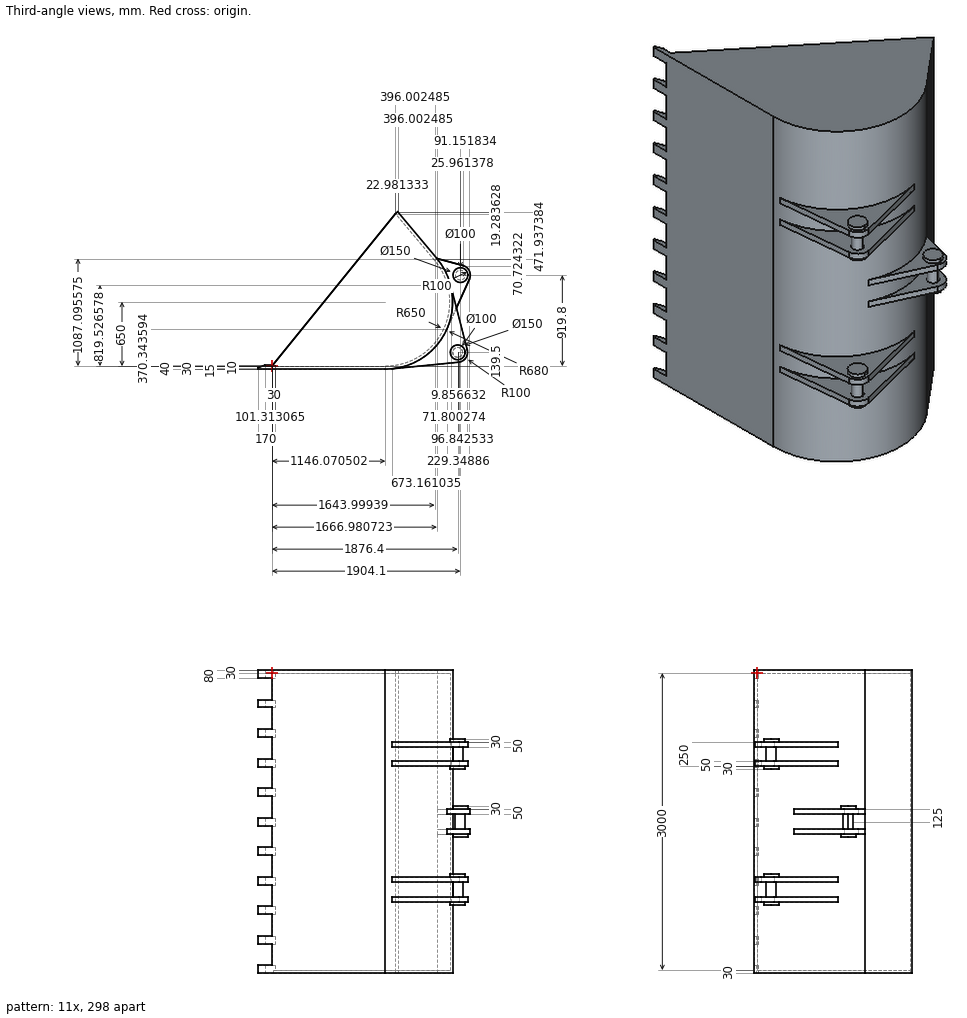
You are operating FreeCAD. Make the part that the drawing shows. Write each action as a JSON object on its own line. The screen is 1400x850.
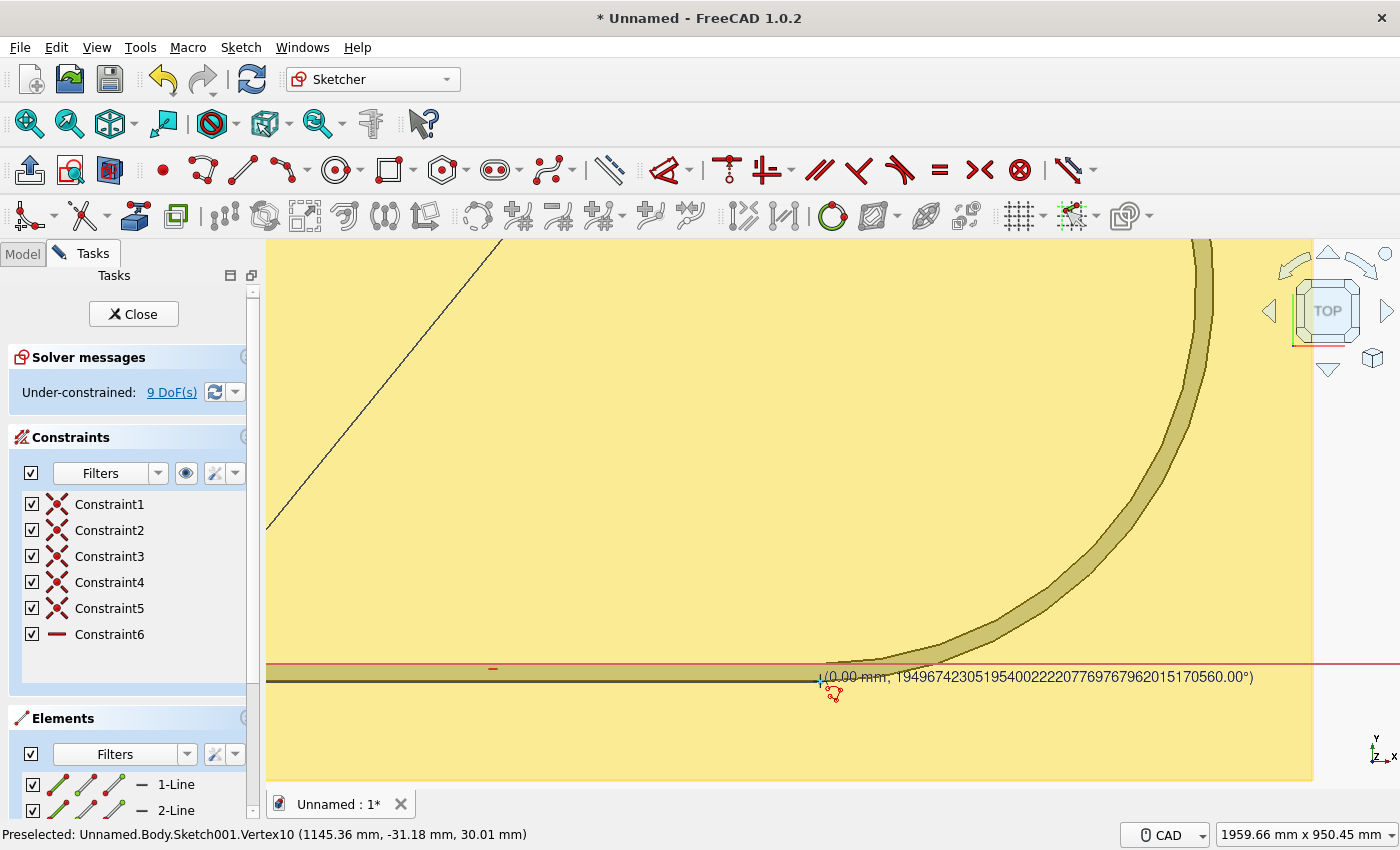
{"action": "left_click", "coordinate": [284, 170]}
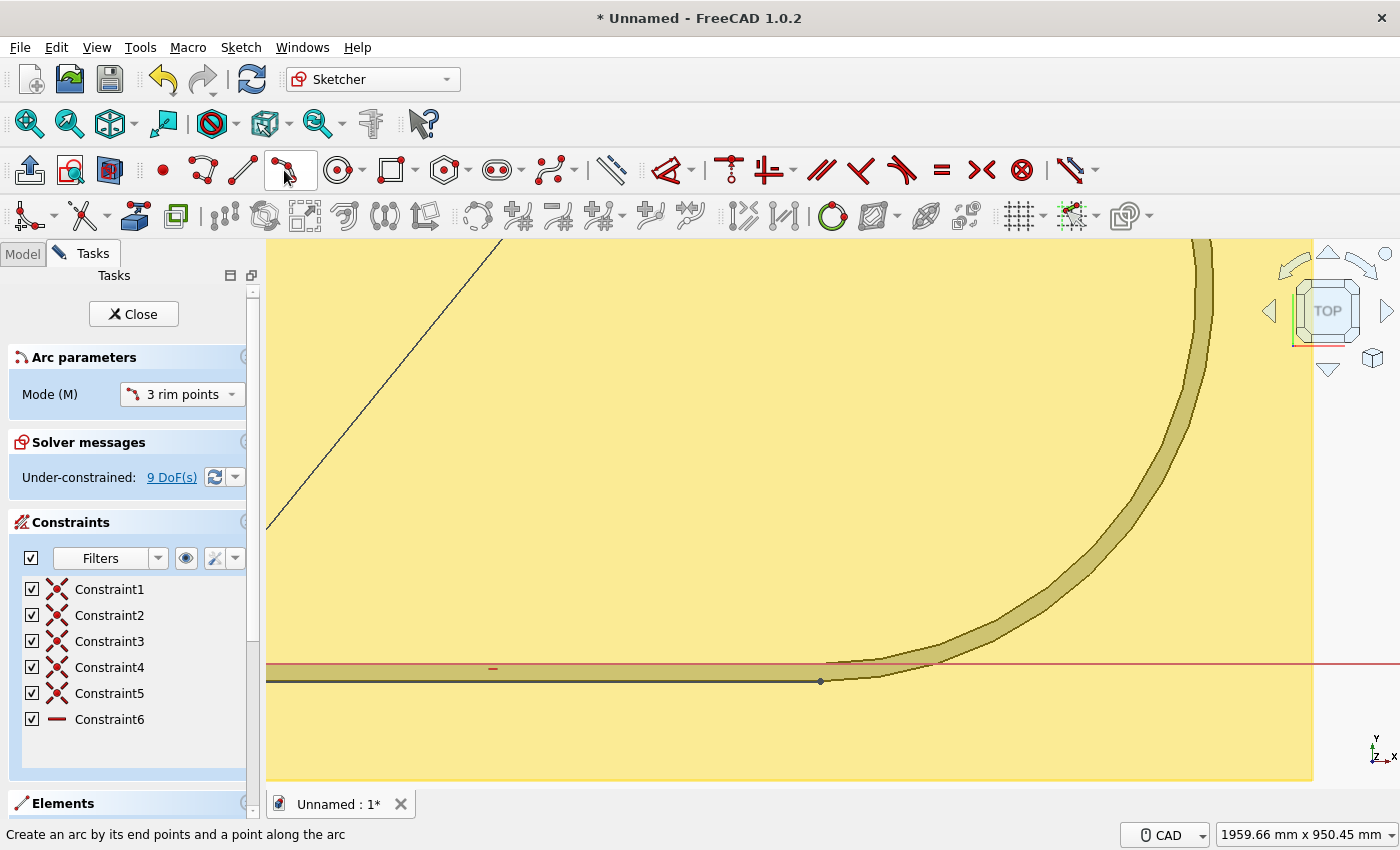
{"action": "left_click", "coordinate": [820, 682]}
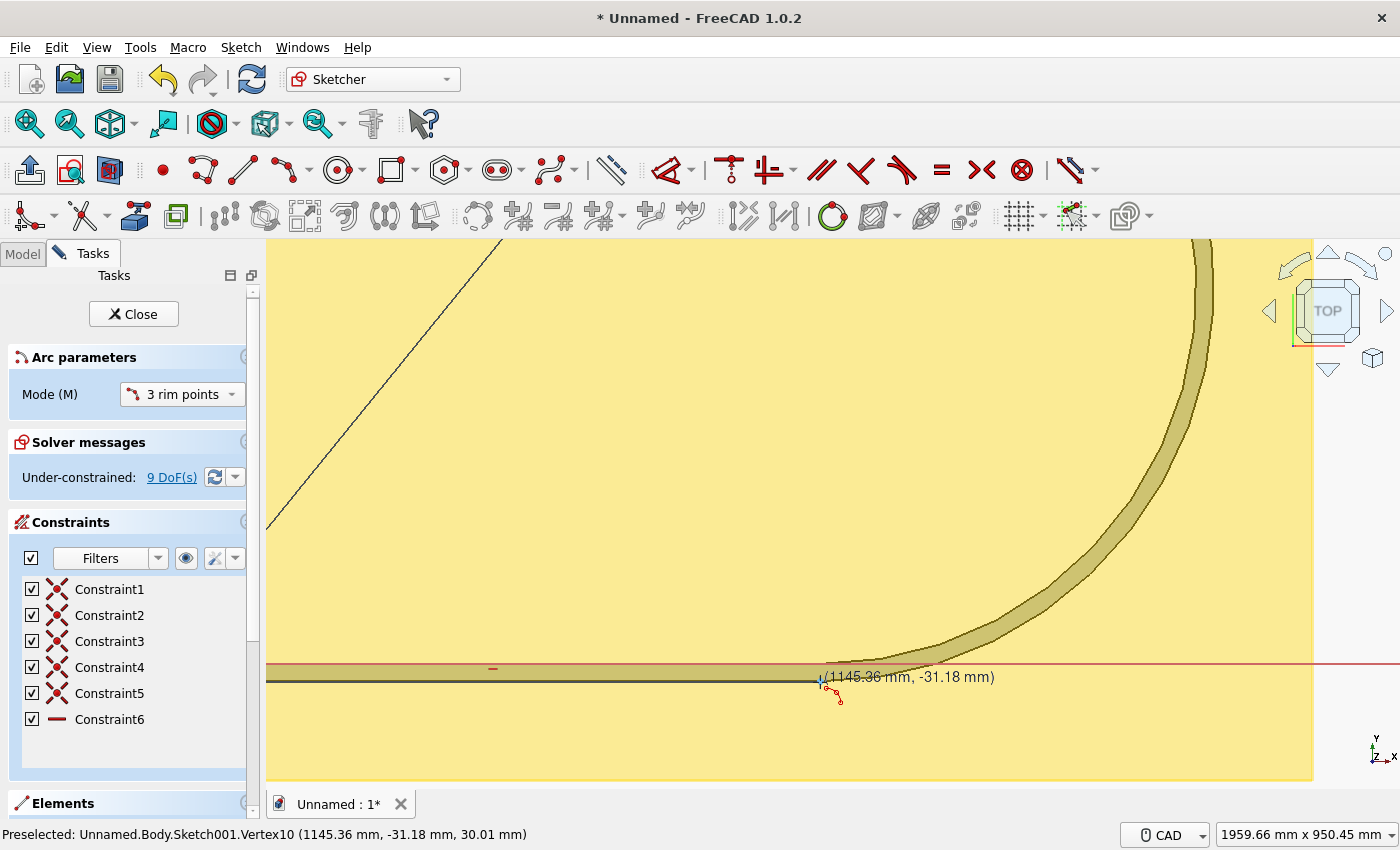
{"action": "scroll", "coordinate": [821, 684], "scroll_direction": "down", "scroll_amount": 5}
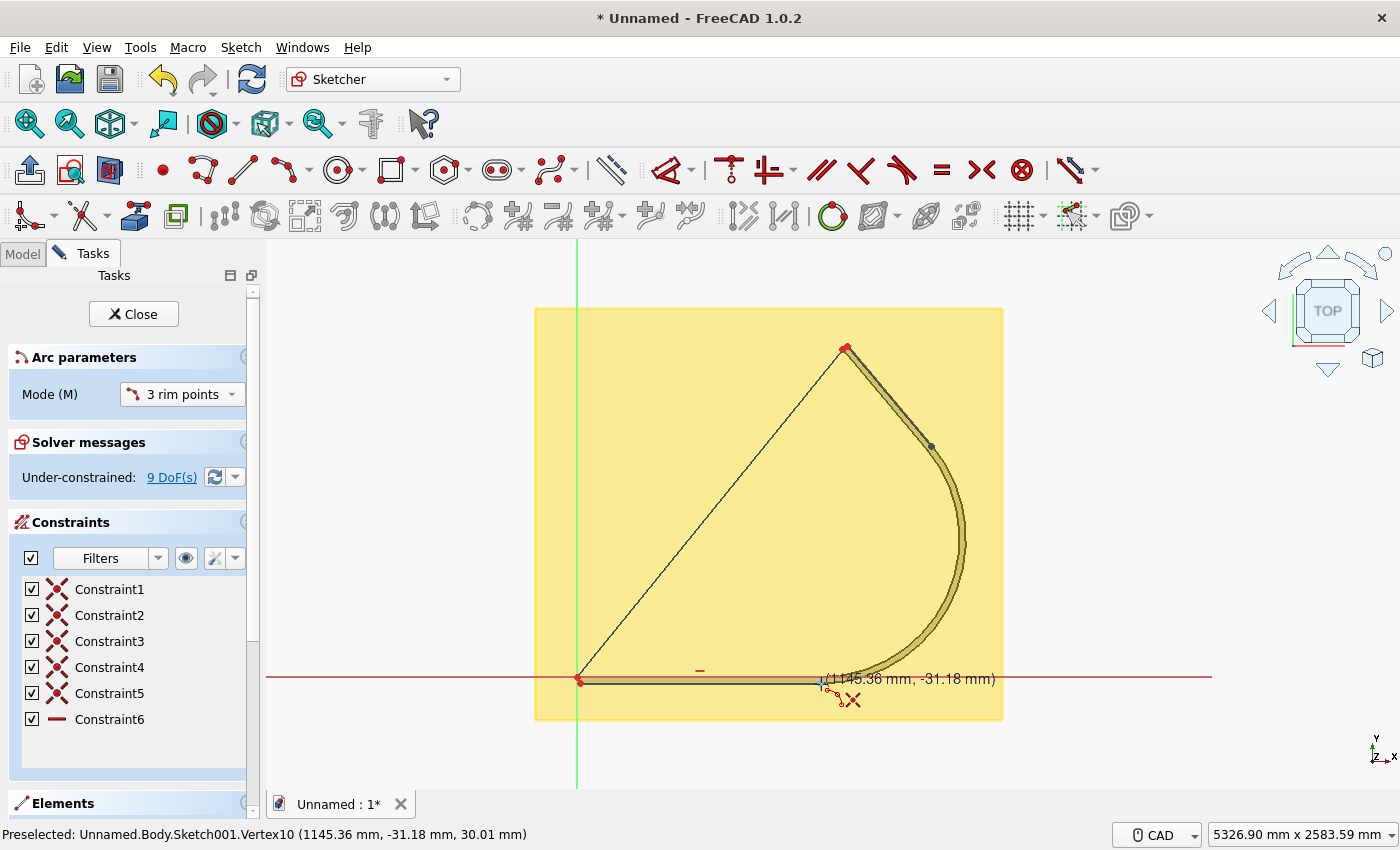
{"action": "left_click", "coordinate": [932, 447]}
{"action": "left_click", "coordinate": [952, 600]}
{"action": "key", "text": "Escape"}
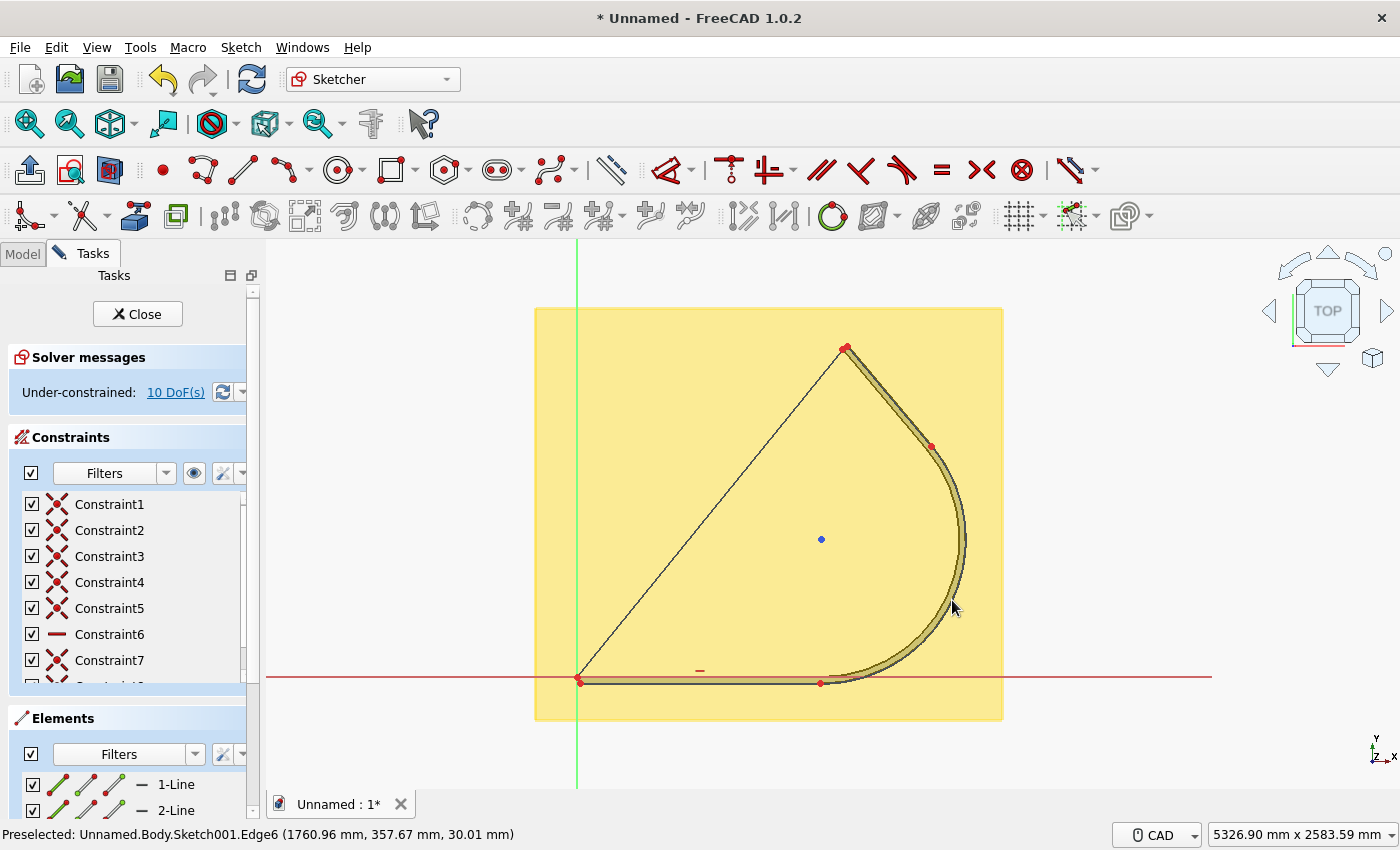
{"action": "scroll", "coordinate": [579, 680], "scroll_direction": "up", "scroll_amount": 7}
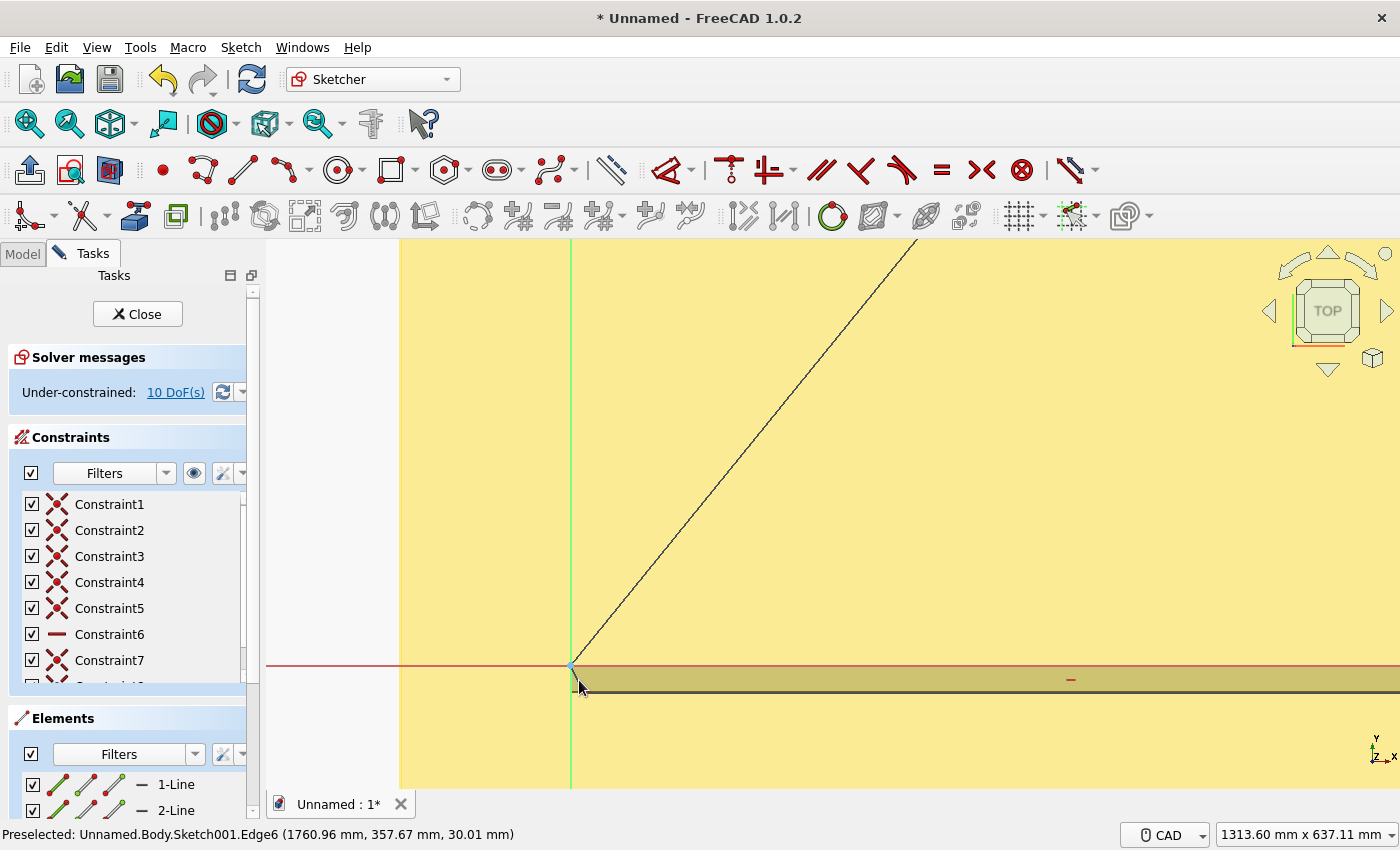
{"action": "left_click", "coordinate": [577, 679]}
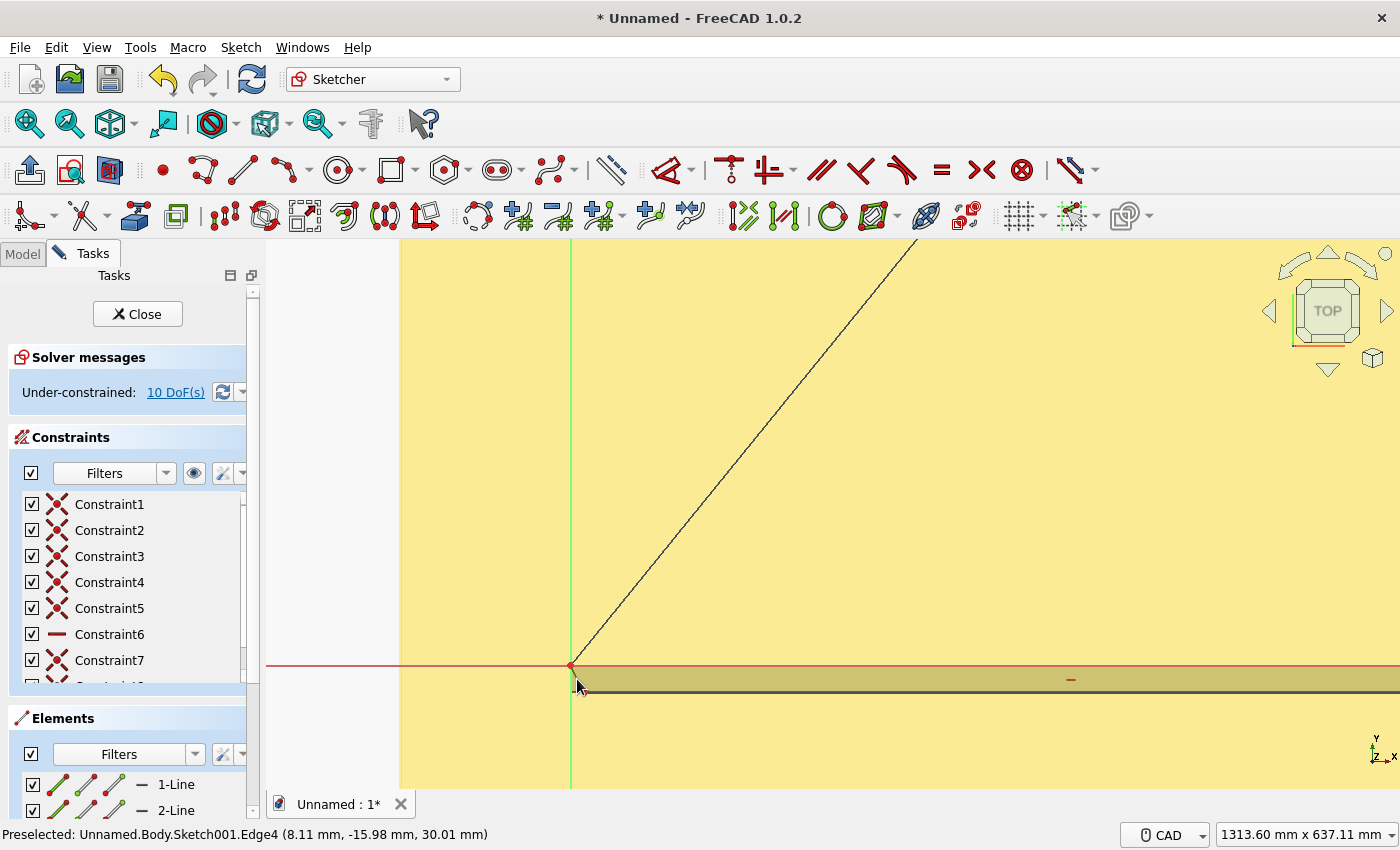
{"action": "key", "text": "v"}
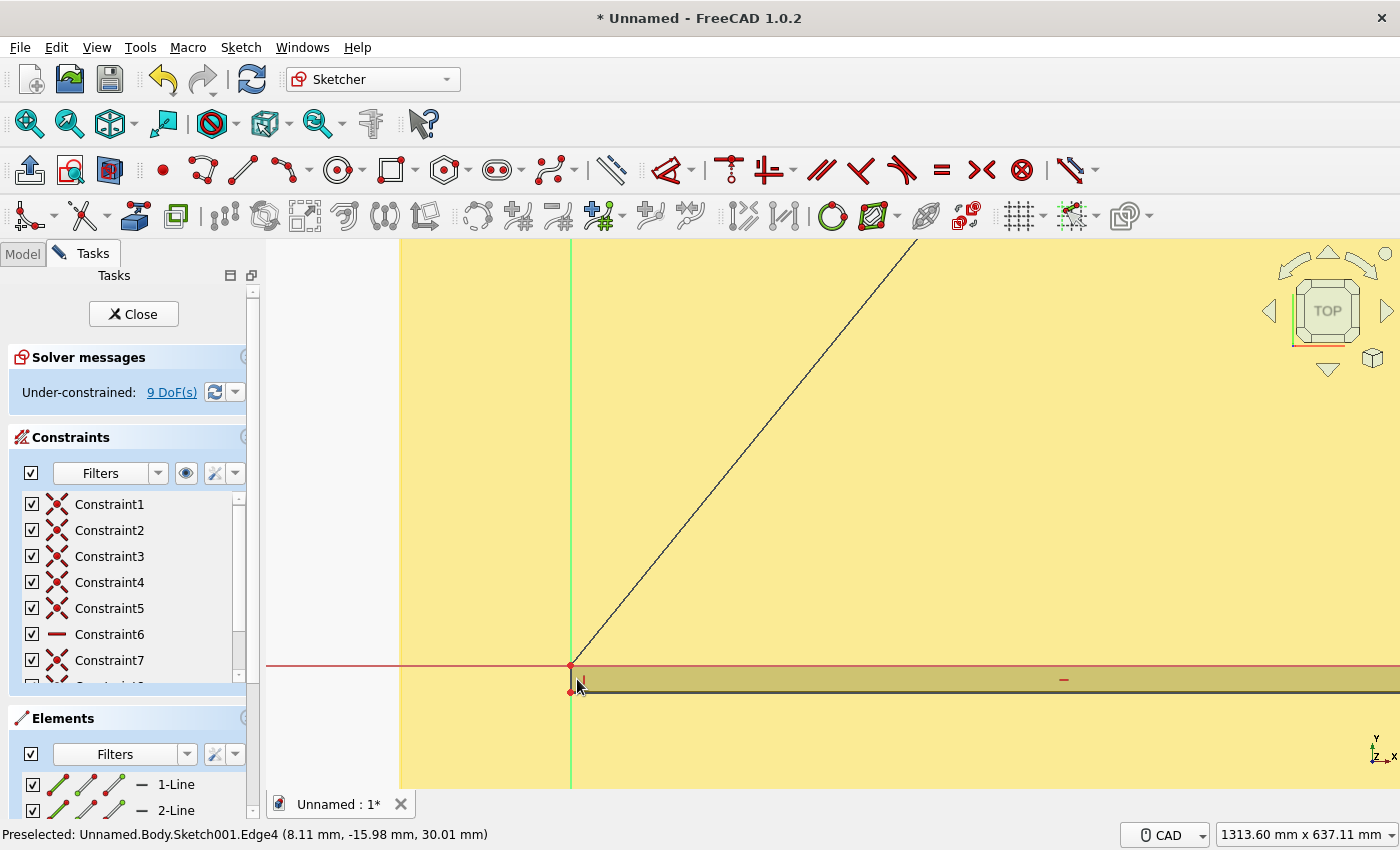
{"action": "left_click", "coordinate": [666, 170]}